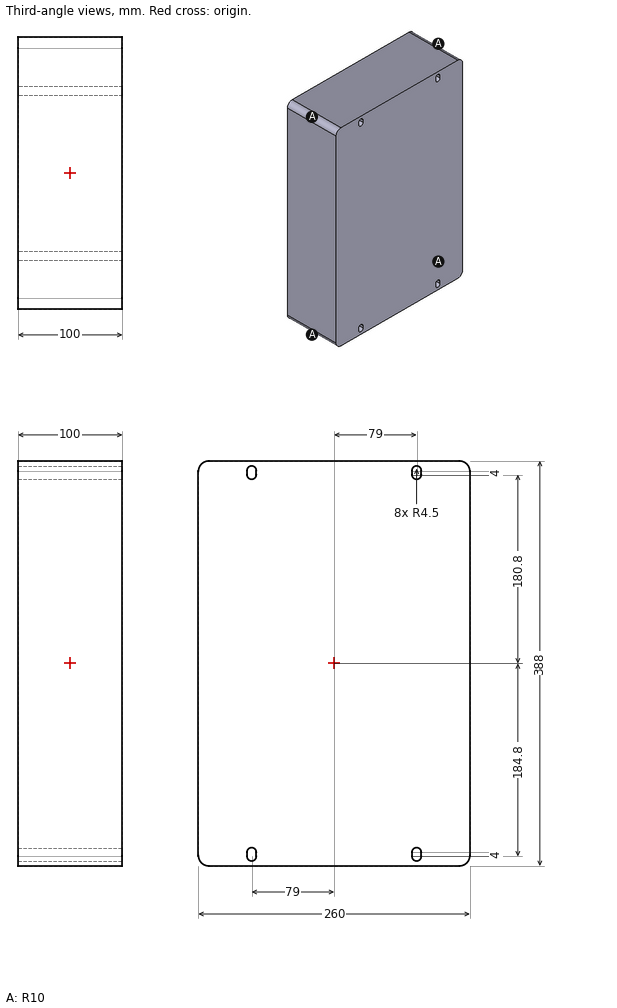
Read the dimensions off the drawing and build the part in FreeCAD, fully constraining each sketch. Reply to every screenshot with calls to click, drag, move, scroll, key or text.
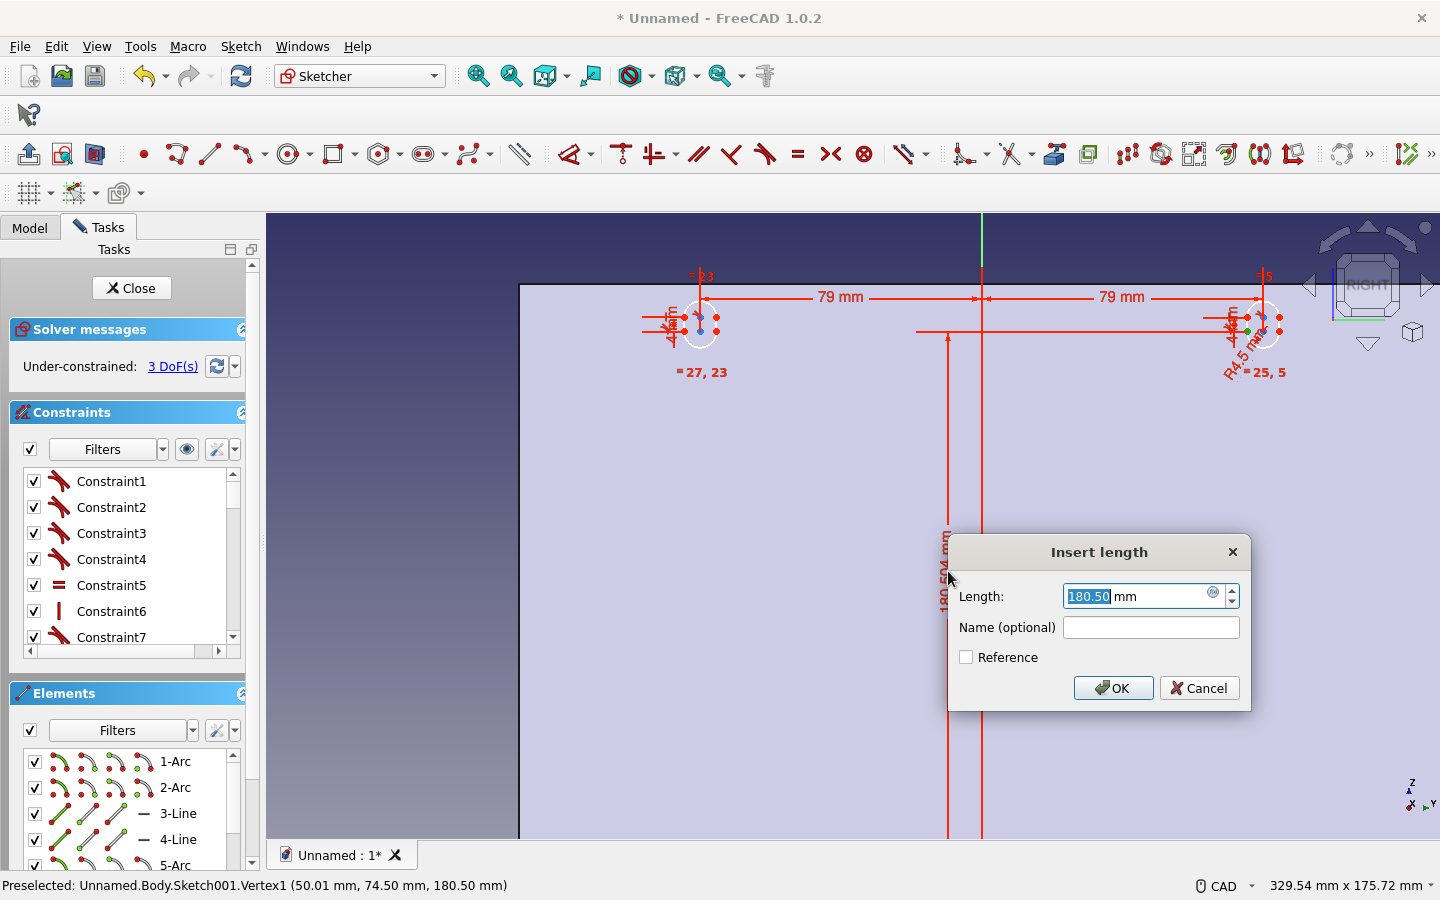
text(180.8)
key(Return)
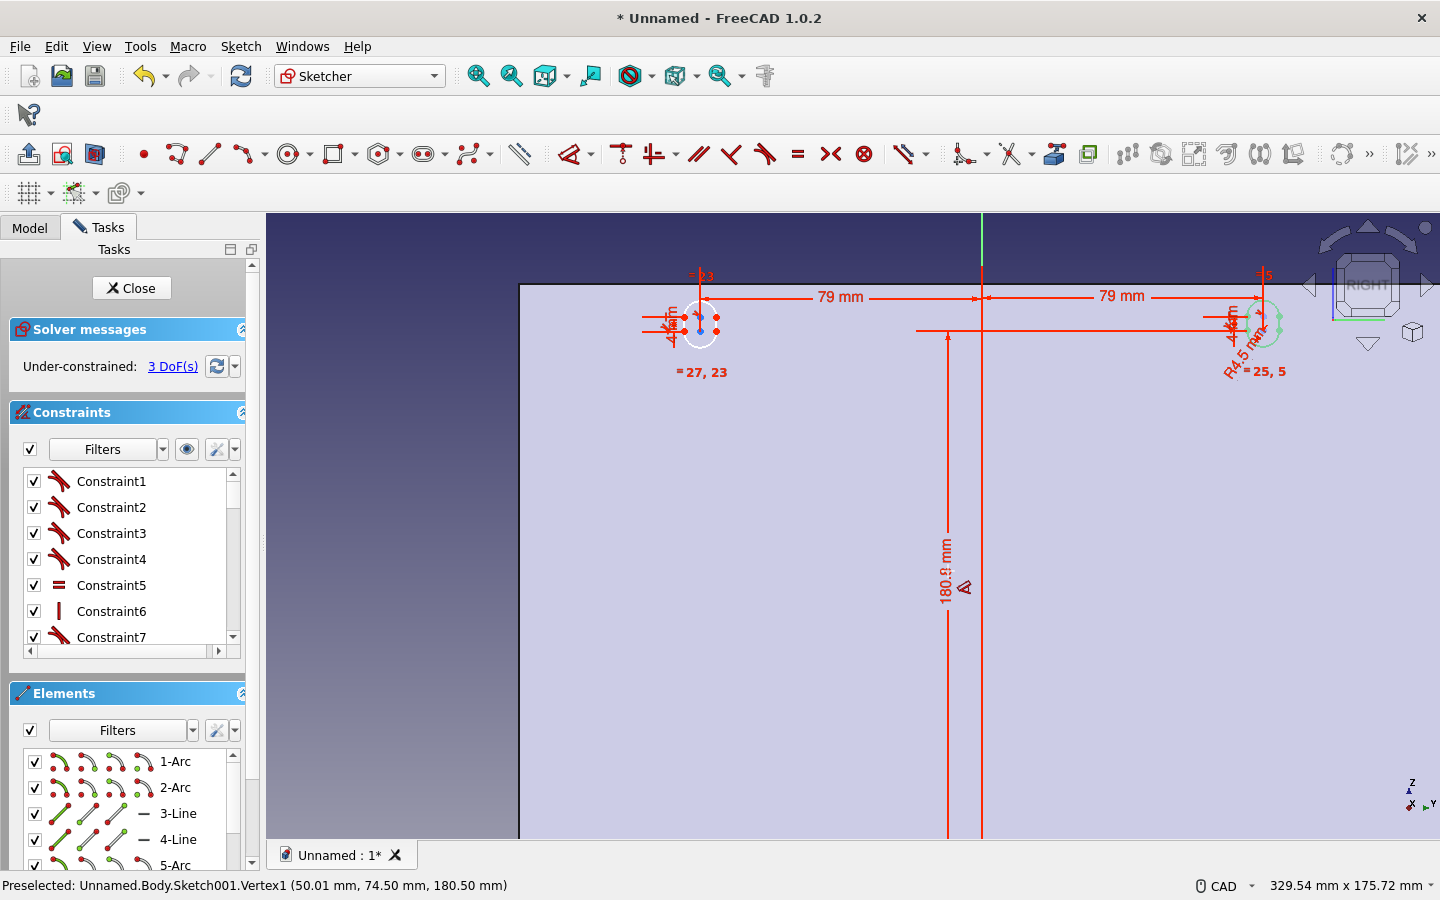
scroll(700, 333, down, 6)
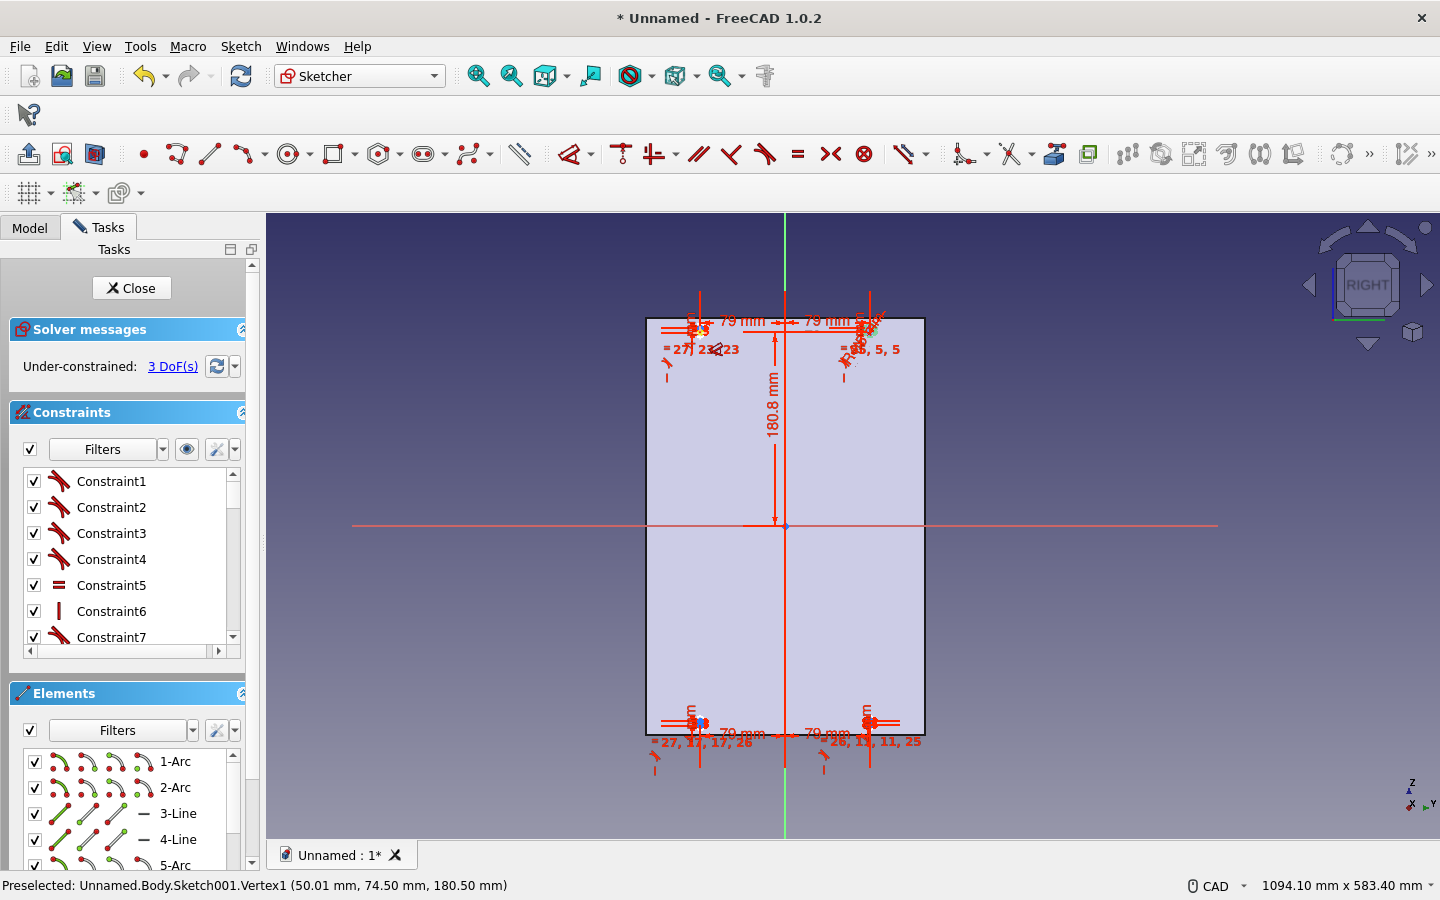
scroll(865, 725, up, 6)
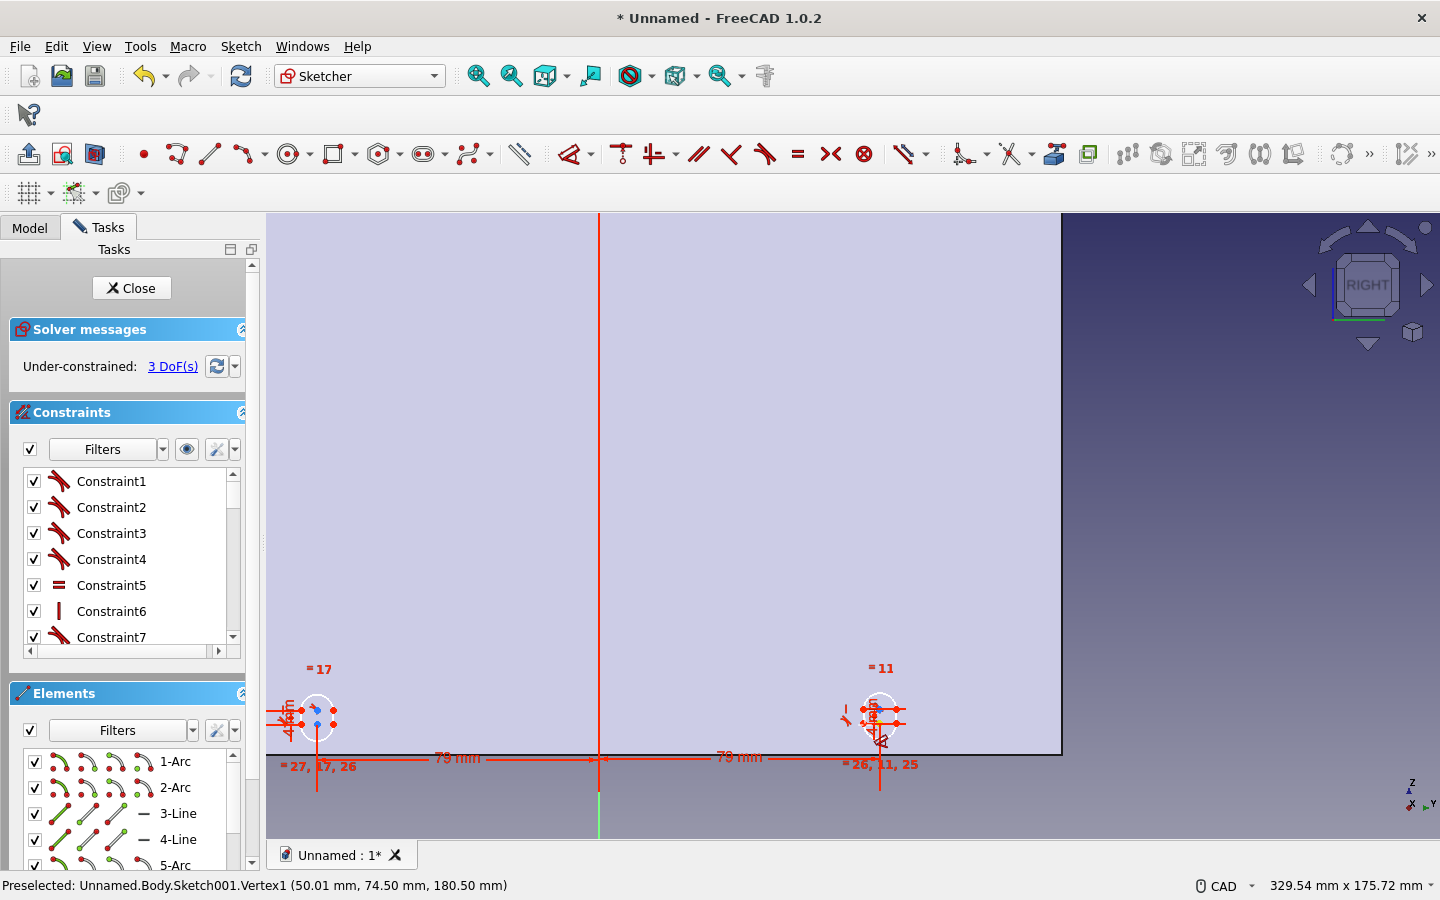
click(864, 724)
click(898, 482)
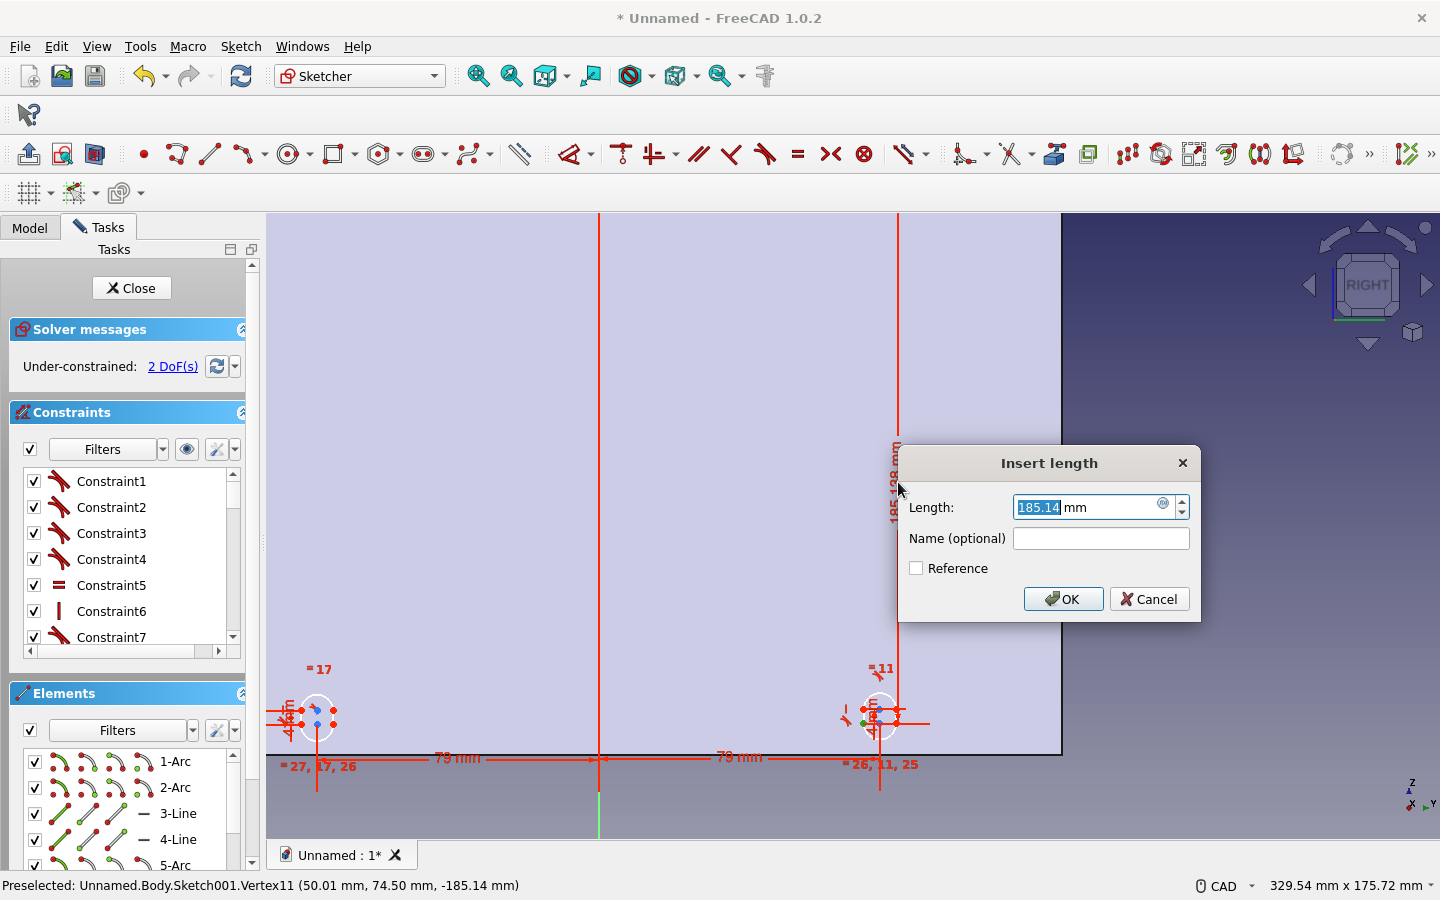
text(184.8)
key(Return)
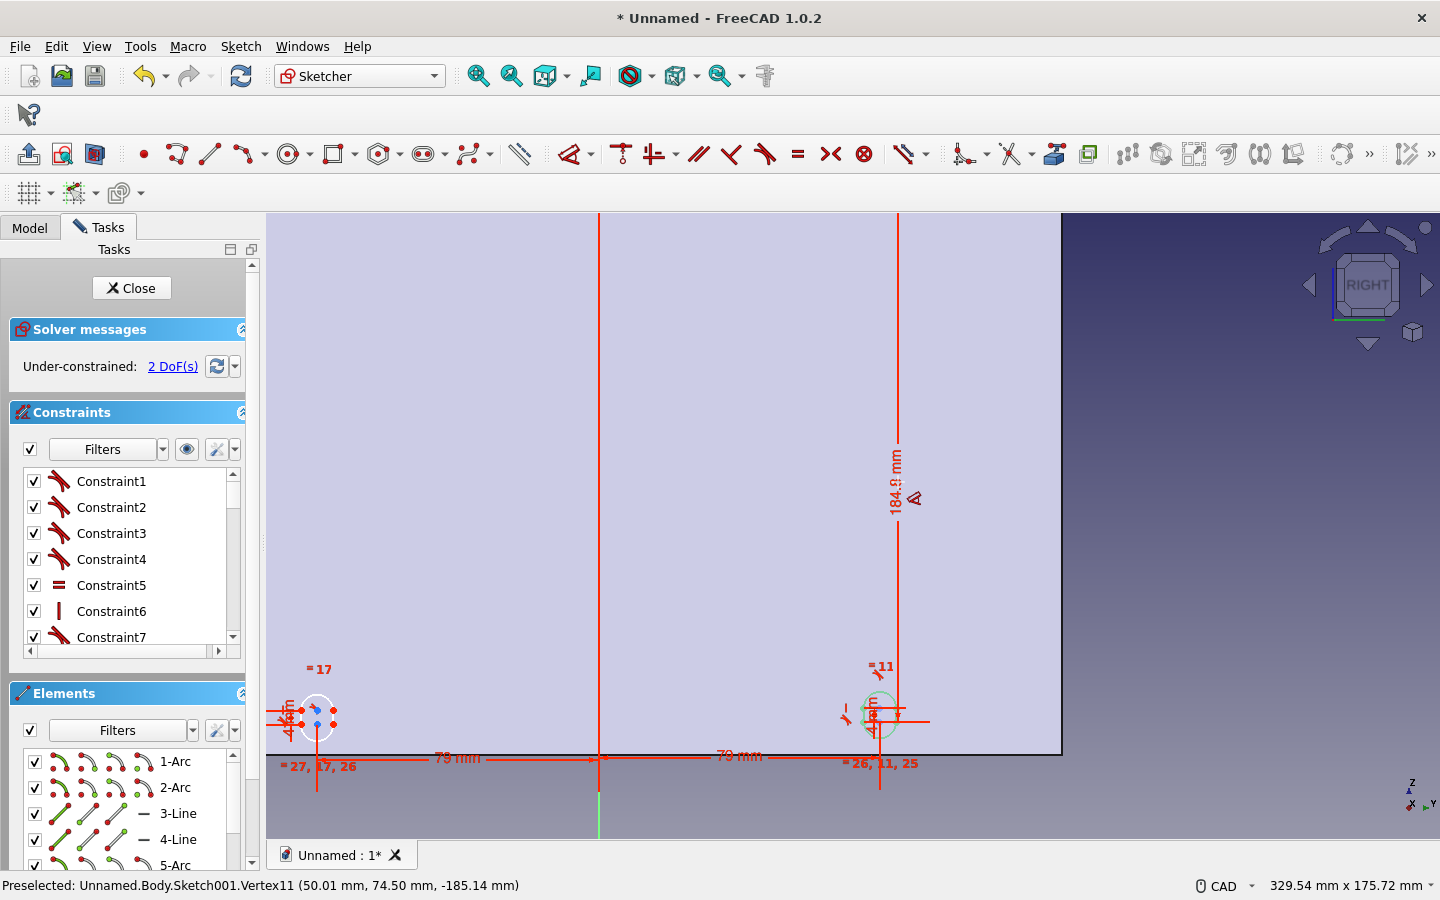
click(301, 725)
click(633, 483)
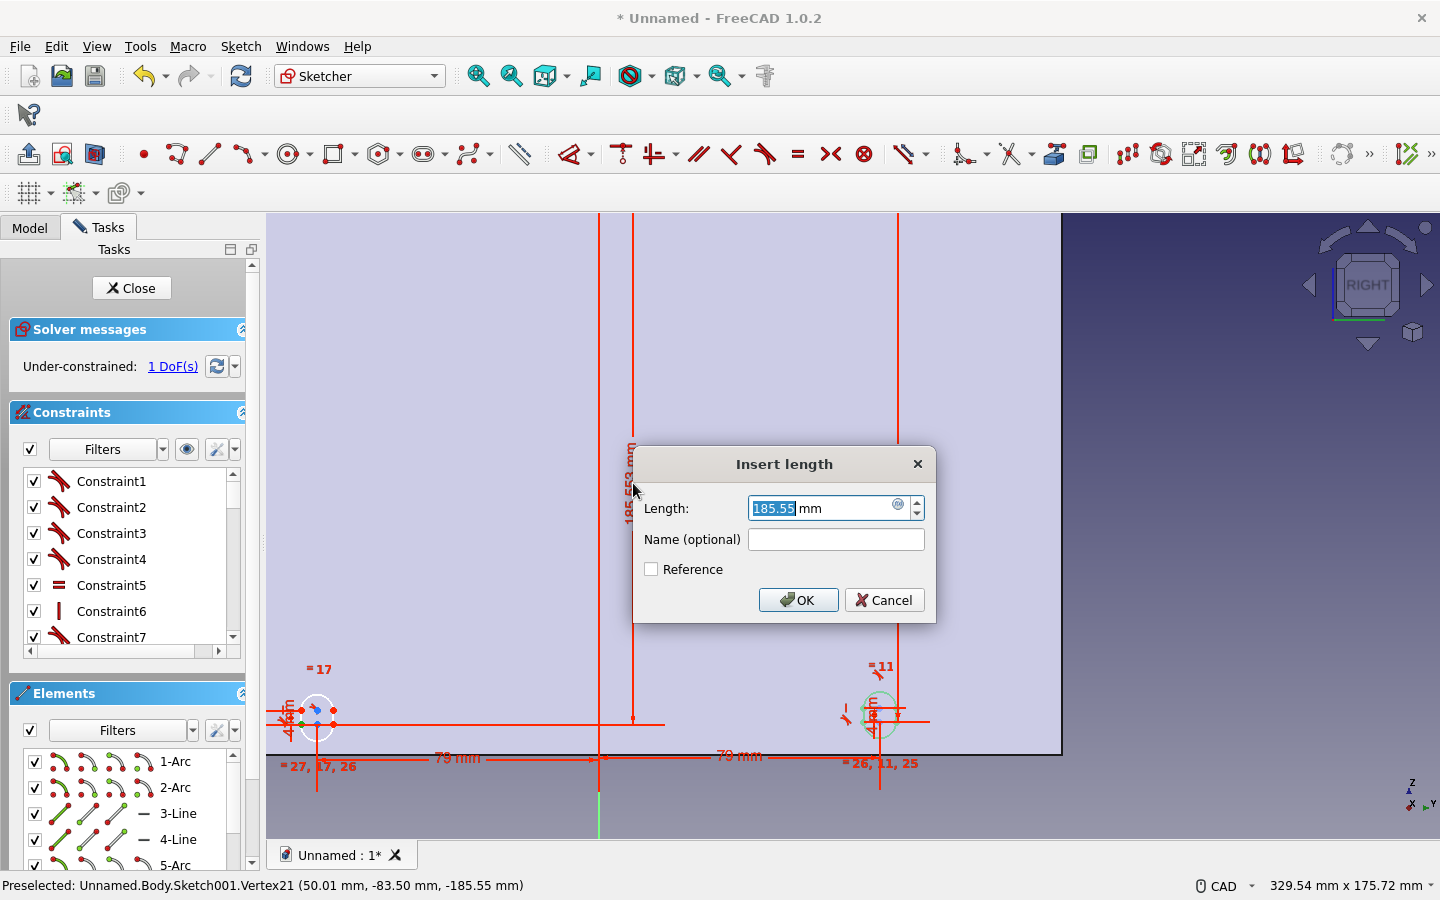
text(184.8)
key(Return)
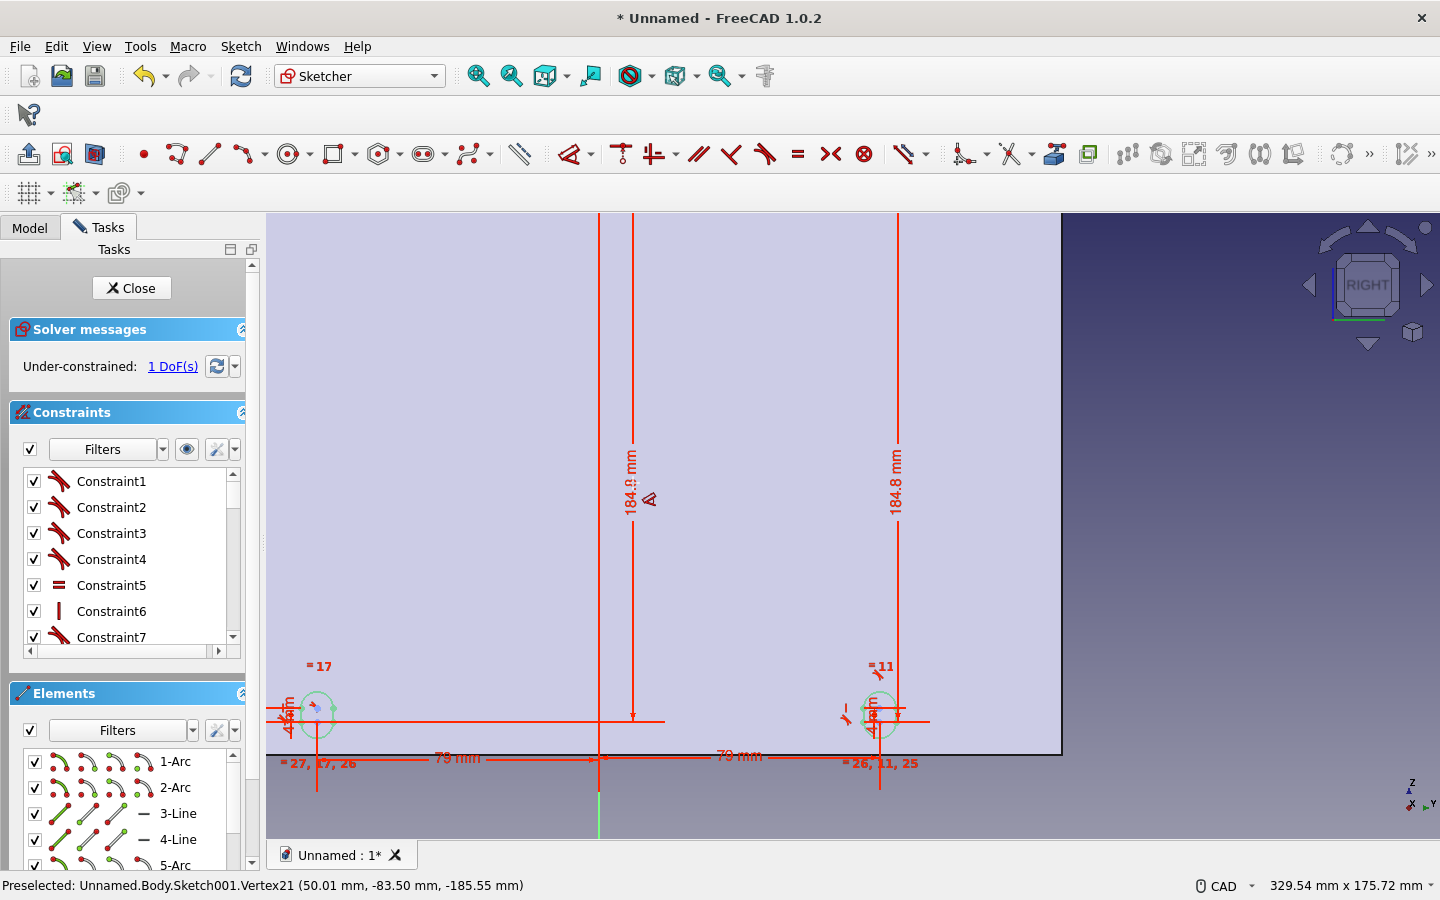
scroll(865, 725, down, 6)